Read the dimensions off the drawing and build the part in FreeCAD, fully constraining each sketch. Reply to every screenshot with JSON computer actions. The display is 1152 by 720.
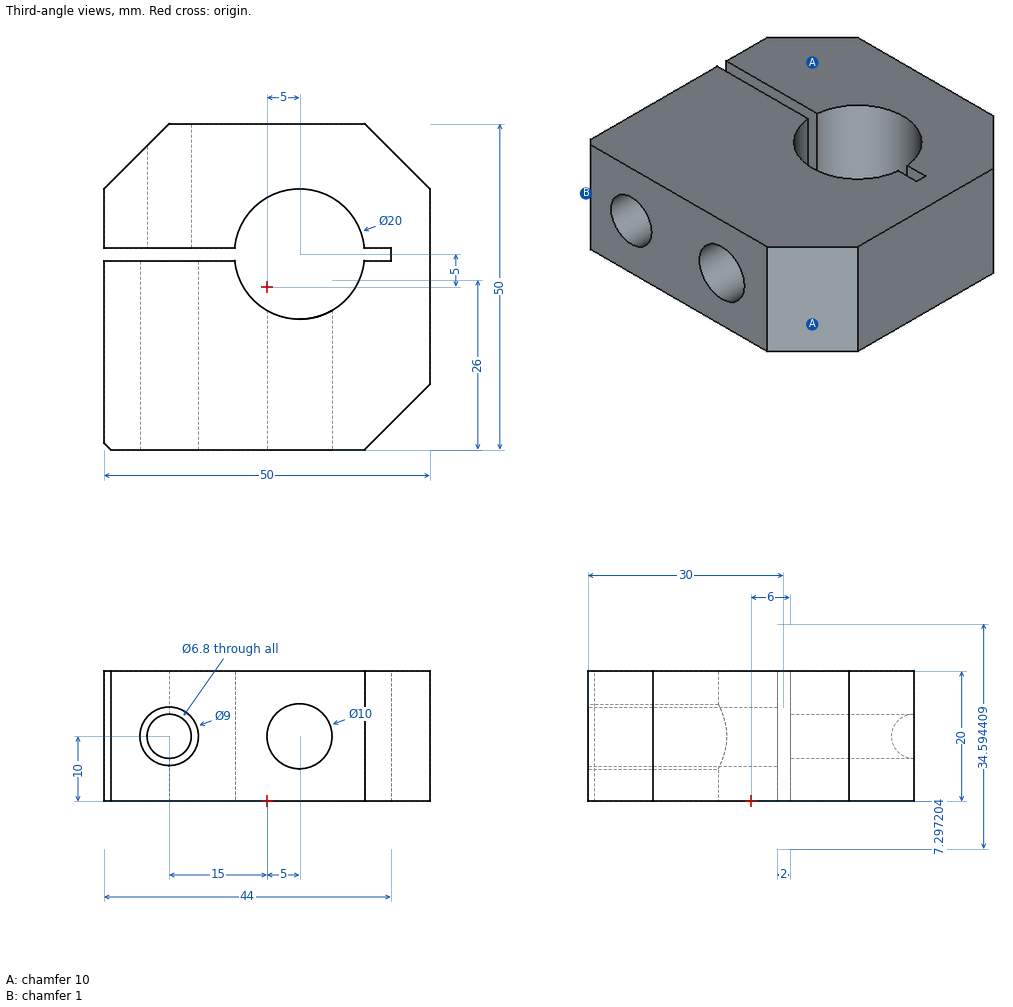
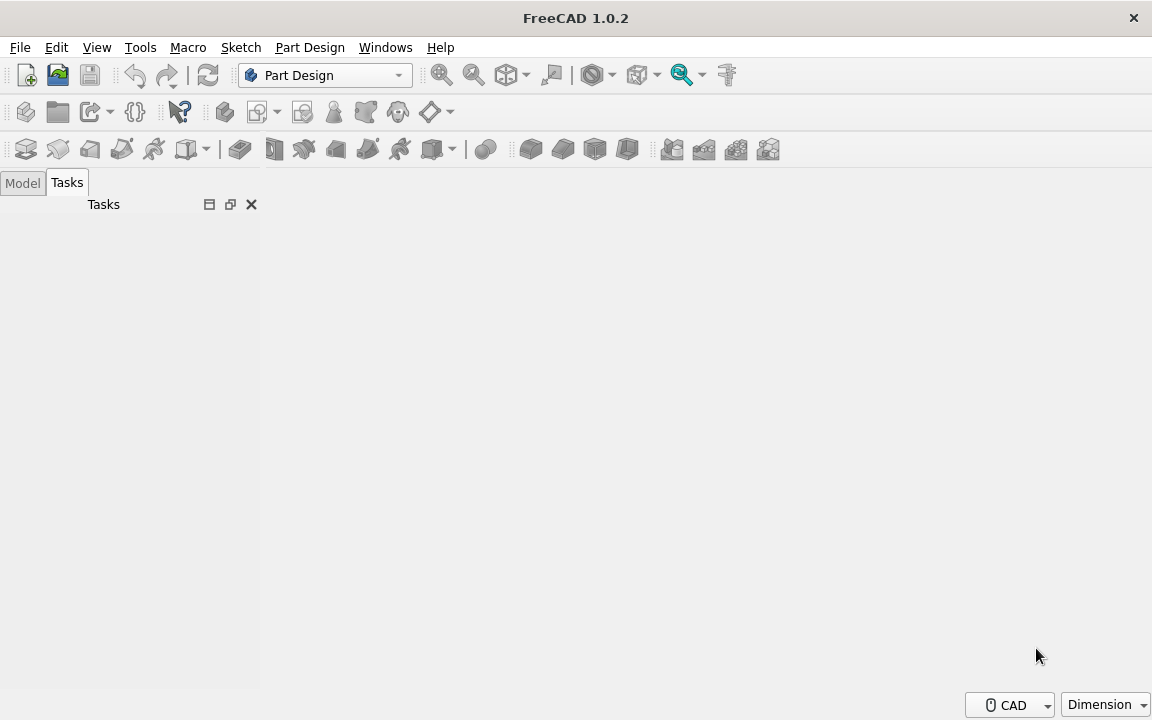
{"action": "left_click", "coordinate": [26, 76]}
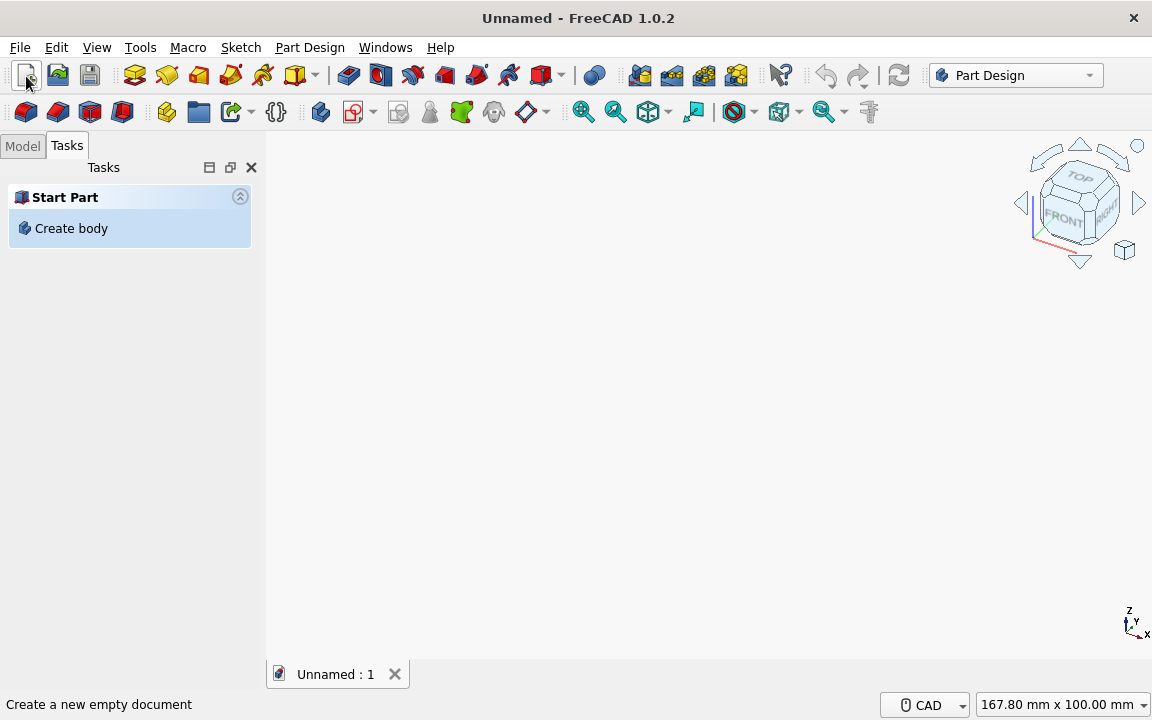
{"action": "left_click", "coordinate": [354, 112]}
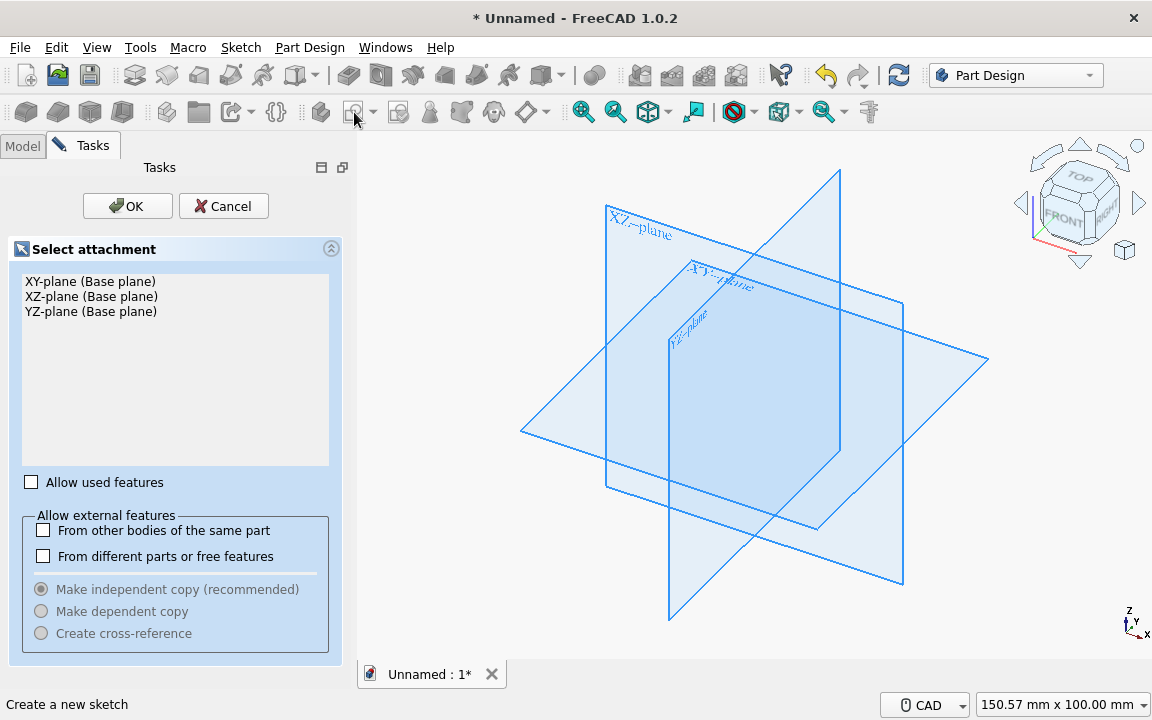
{"action": "left_click", "coordinate": [82, 282]}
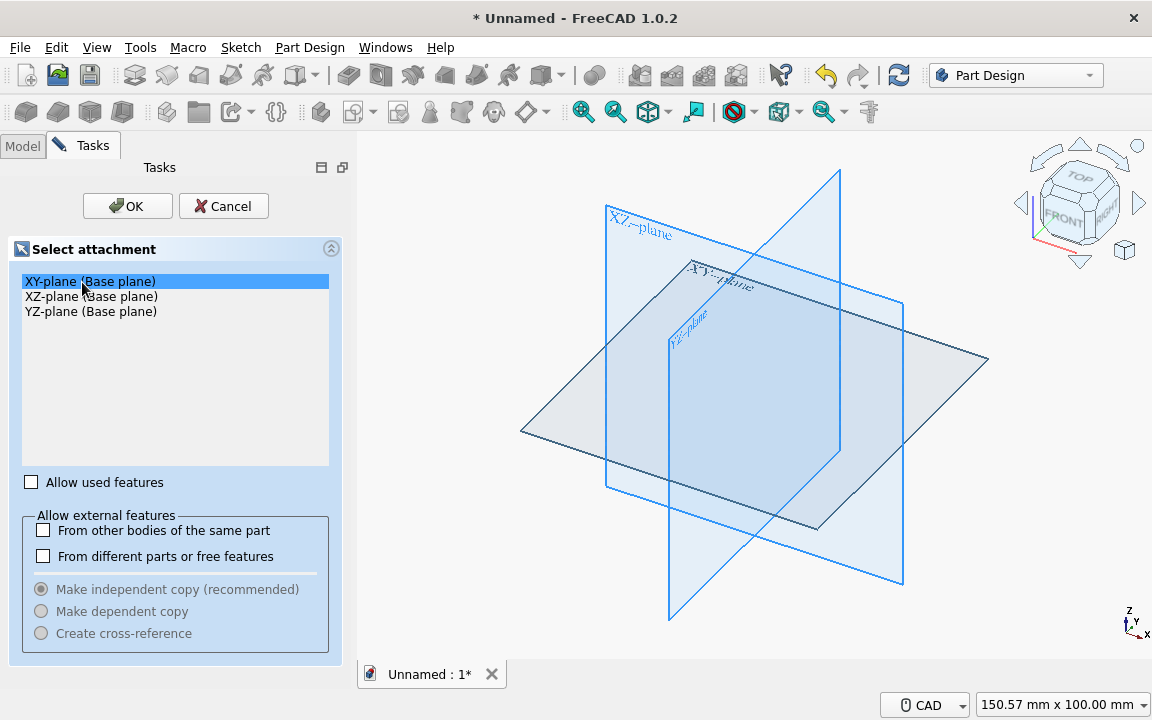
{"action": "left_click", "coordinate": [128, 206]}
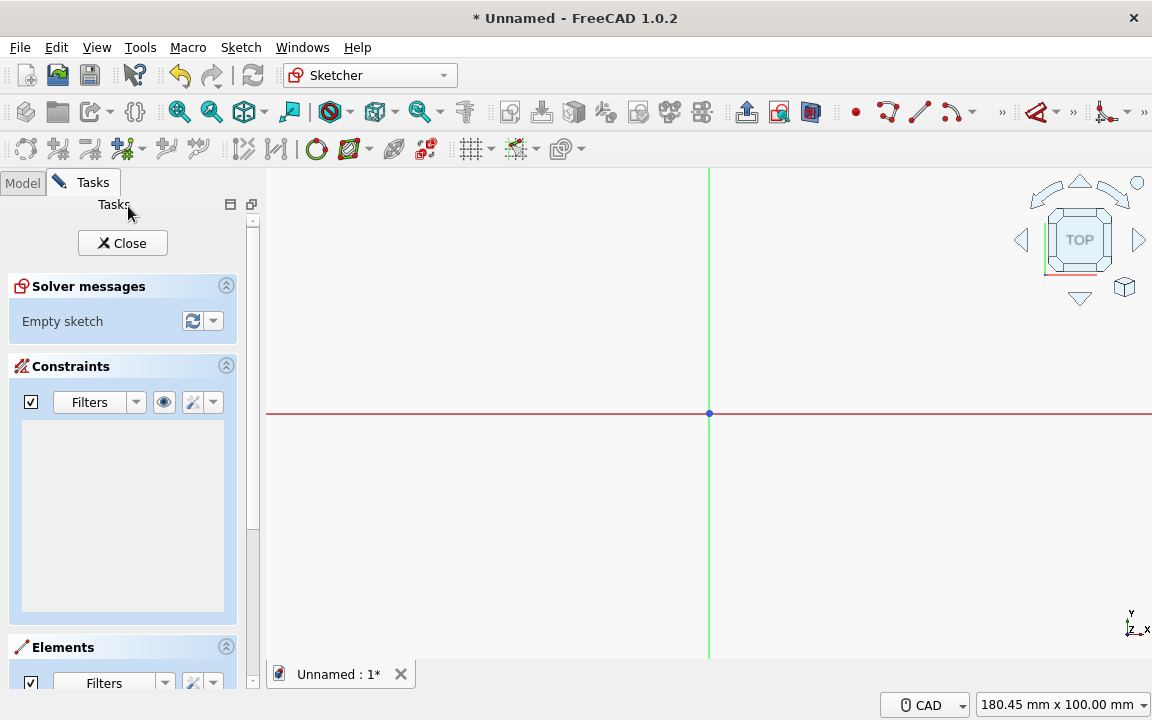
{"action": "key", "text": "g v"}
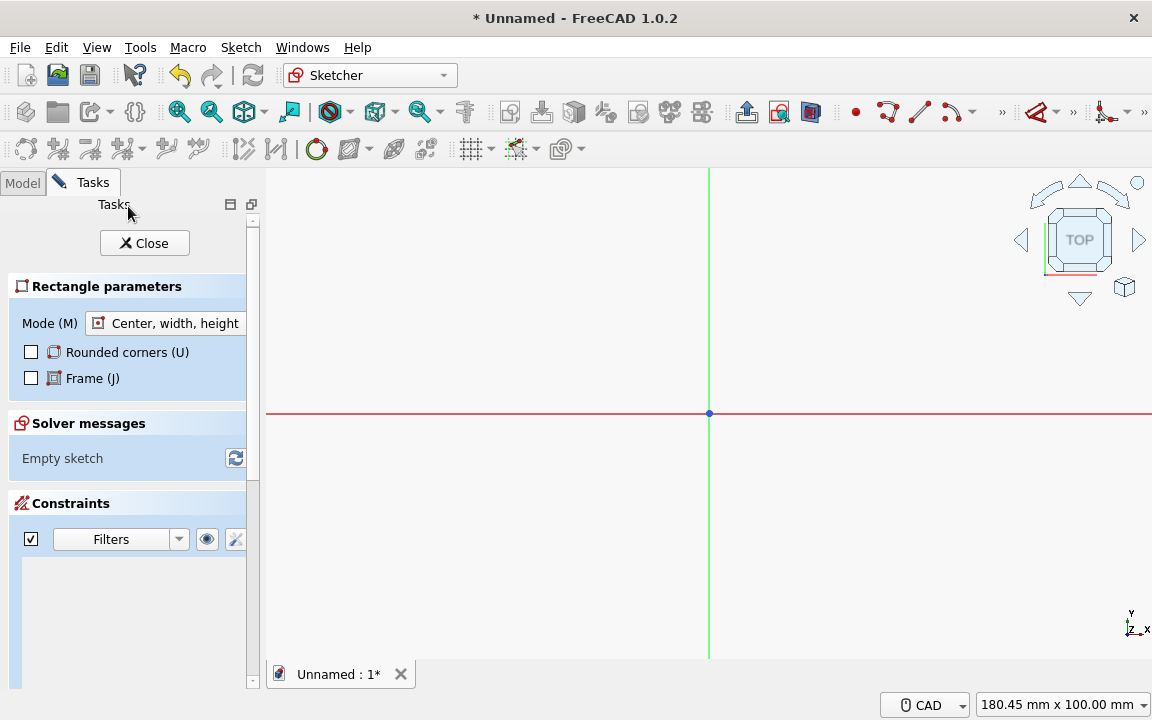
{"action": "left_click", "coordinate": [709, 414]}
{"action": "mouse_move", "coordinate": [832, 291]}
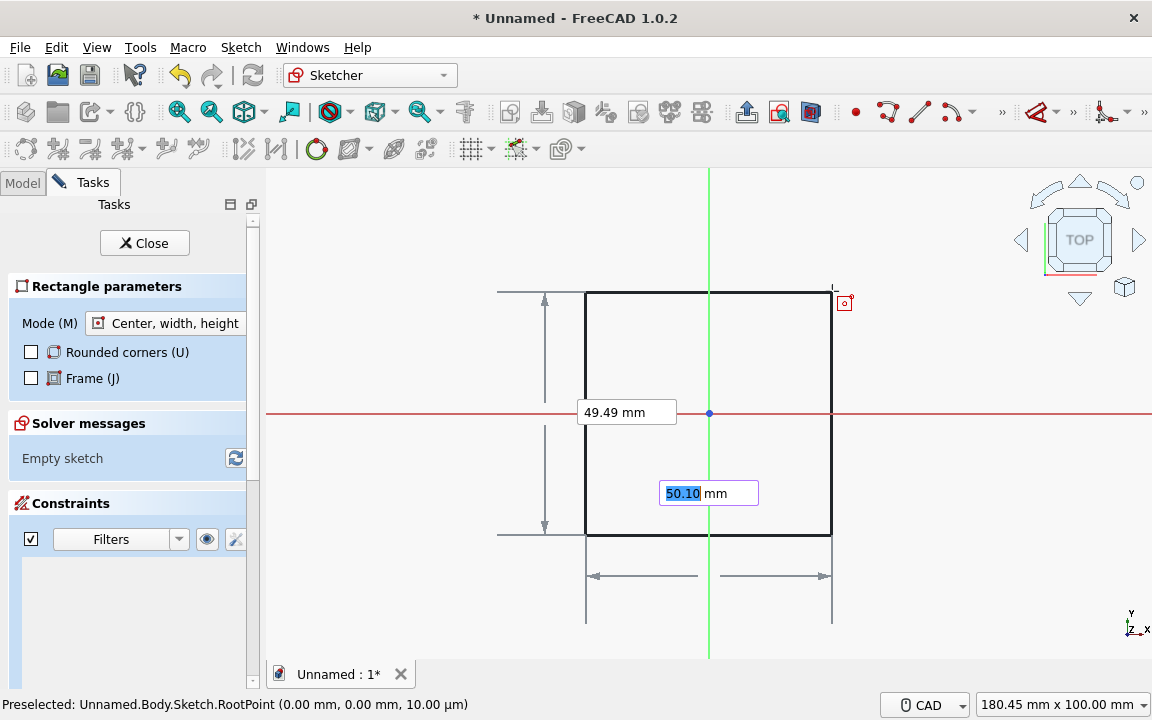
{"action": "type", "text": "50"}
{"action": "key", "text": "Tab"}
{"action": "type", "text": "50"}
{"action": "key", "text": "Return"}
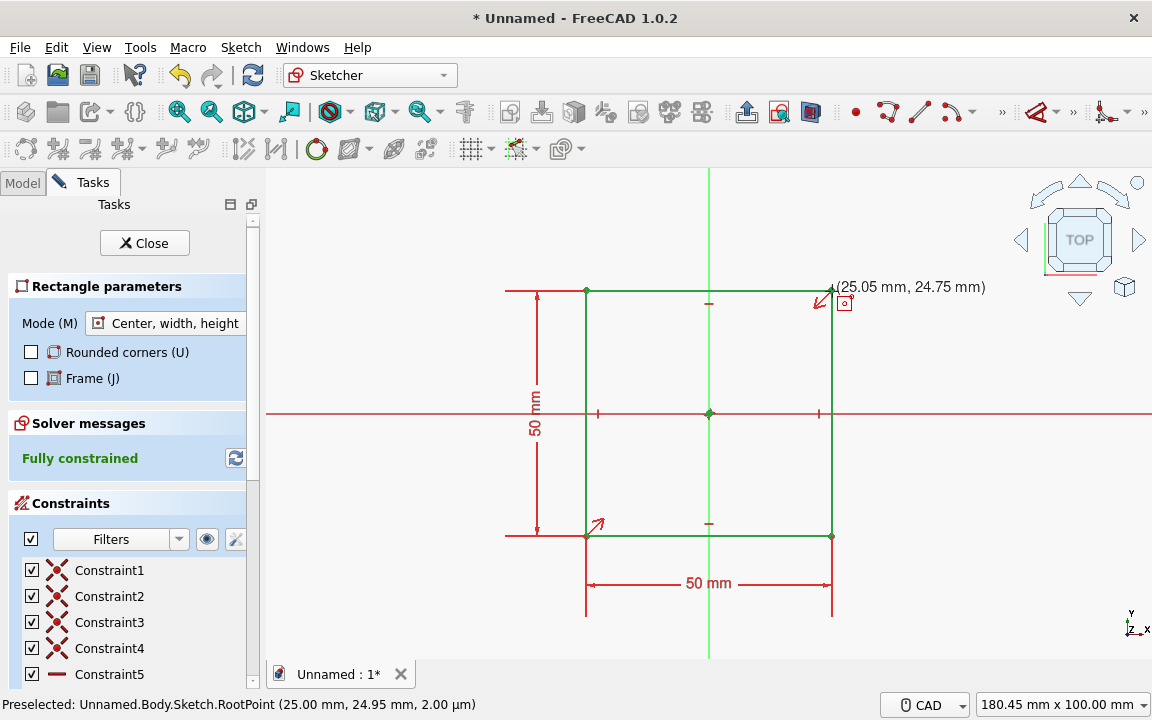
{"action": "key", "text": "g c"}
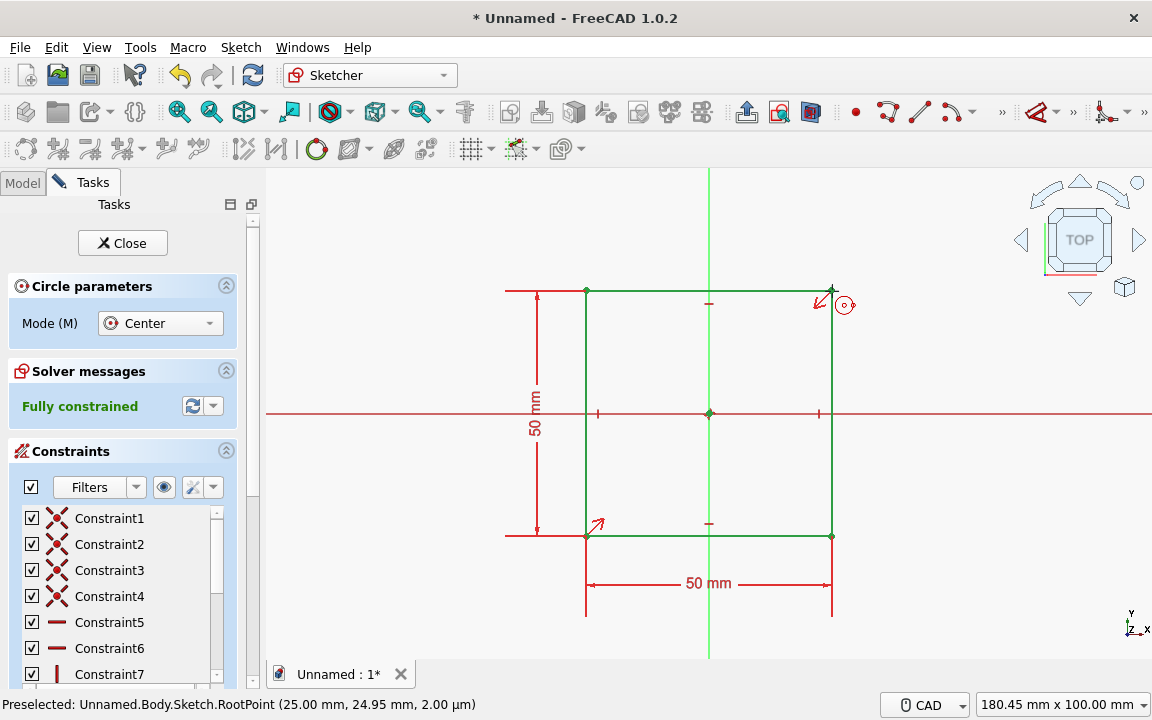
{"action": "left_click", "coordinate": [734, 389]}
{"action": "mouse_move", "coordinate": [768, 354]}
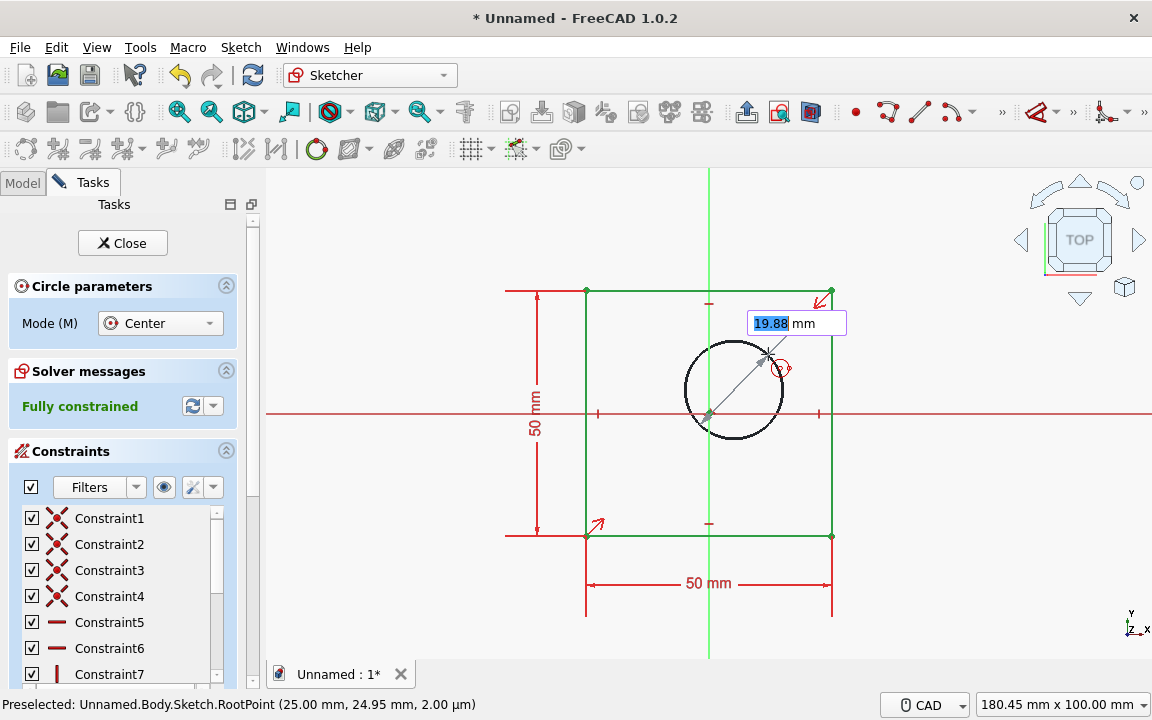
{"action": "type", "text": "20"}
{"action": "key", "text": "Return"}
{"action": "key", "text": "Escape"}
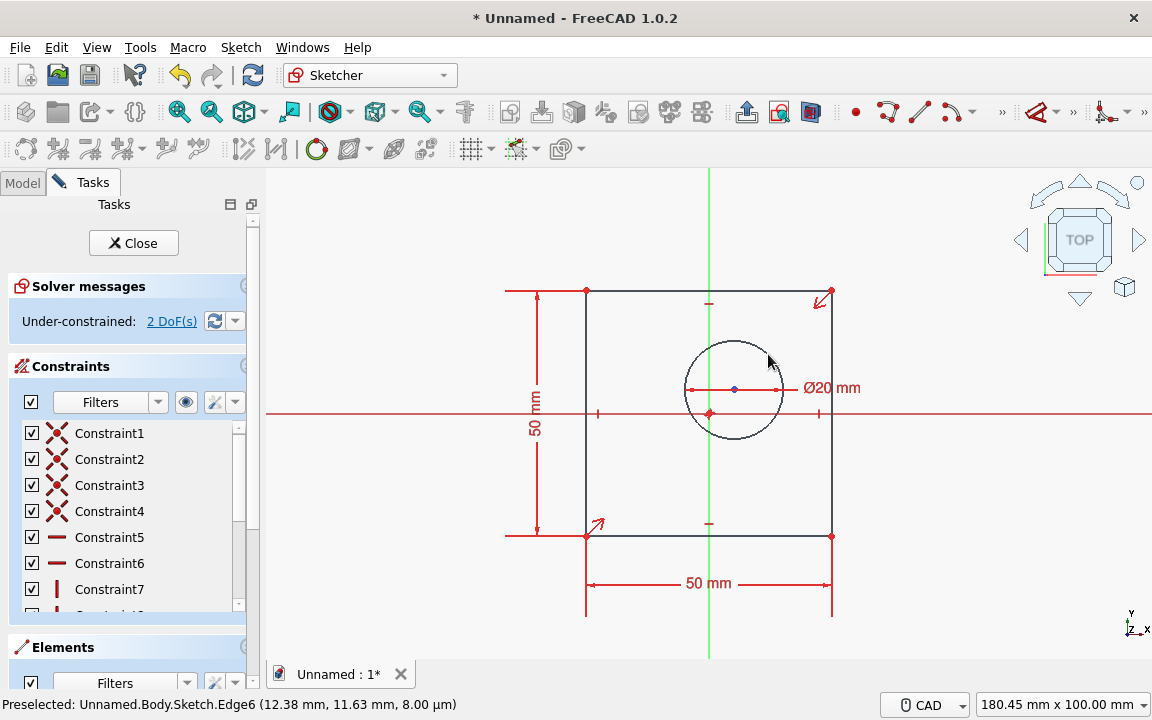
{"action": "left_click", "coordinate": [1036, 112]}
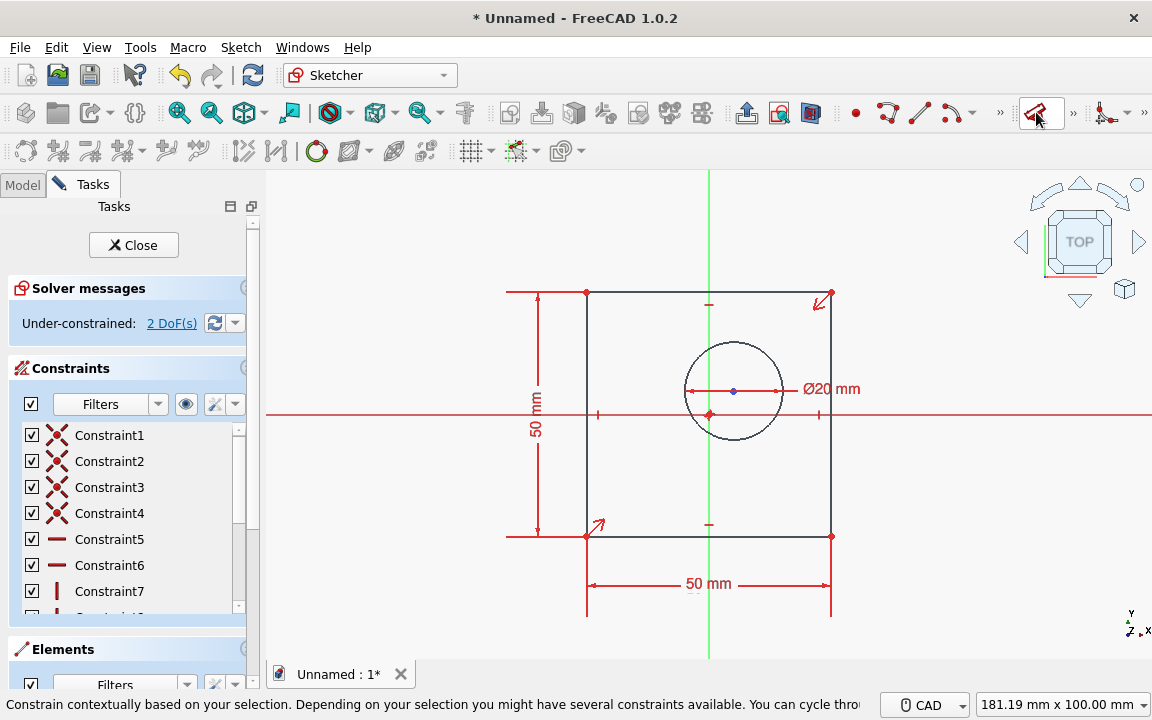
{"action": "scroll", "coordinate": [734, 391], "scroll_direction": "up", "scroll_amount": 3}